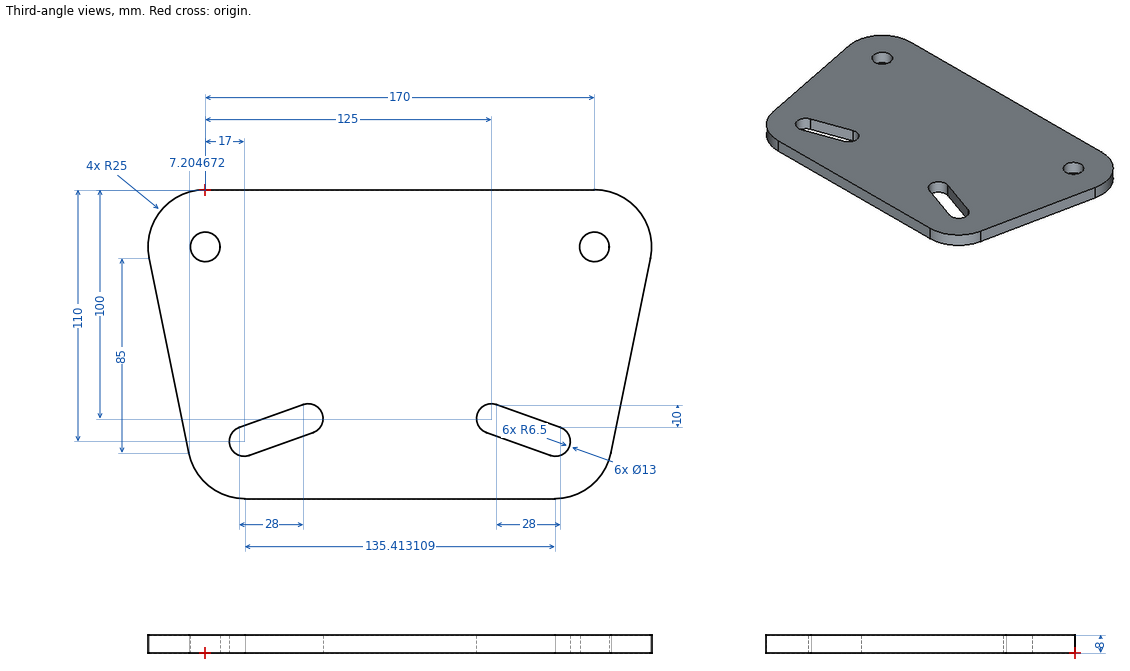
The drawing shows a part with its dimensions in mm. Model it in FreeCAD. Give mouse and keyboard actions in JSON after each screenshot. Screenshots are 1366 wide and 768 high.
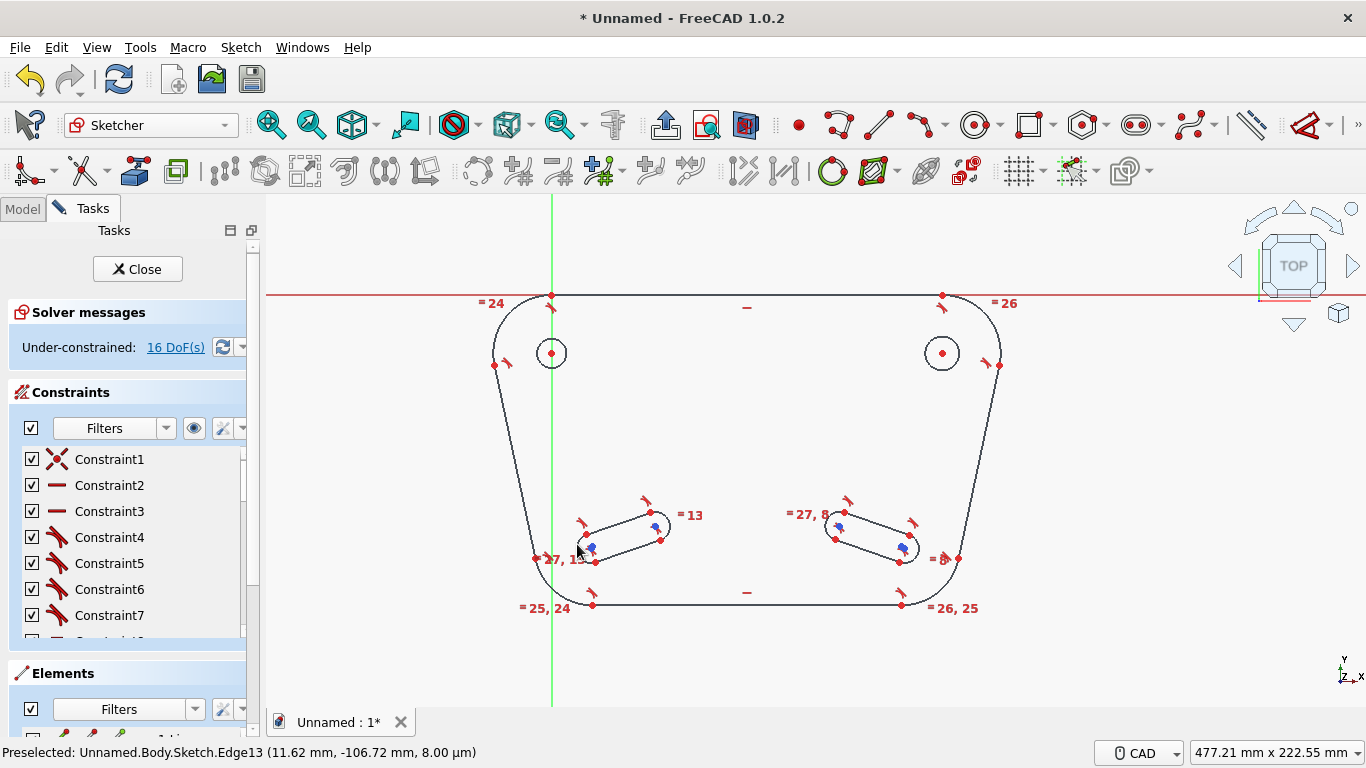
{"action": "left_click", "coordinate": [954, 341]}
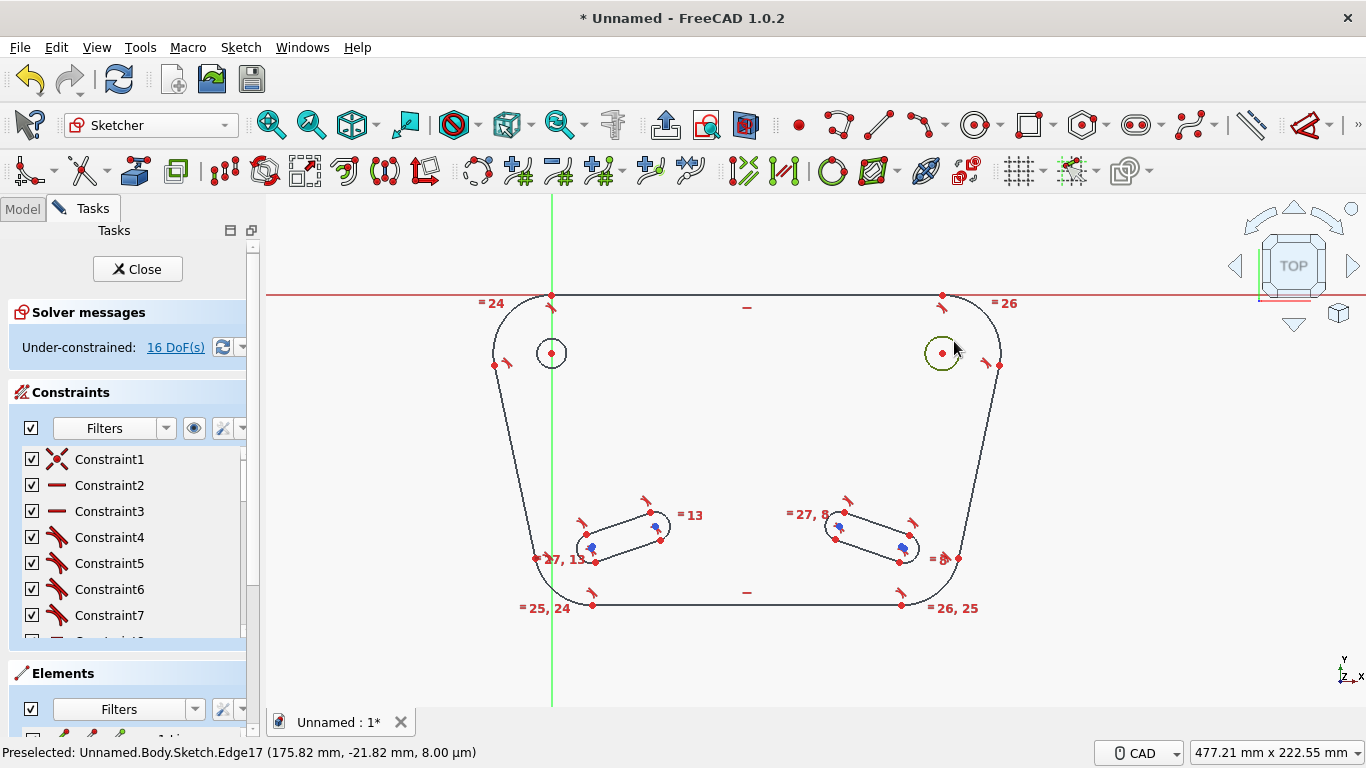
{"action": "scroll", "coordinate": [562, 343], "scroll_direction": "up", "scroll_amount": 2}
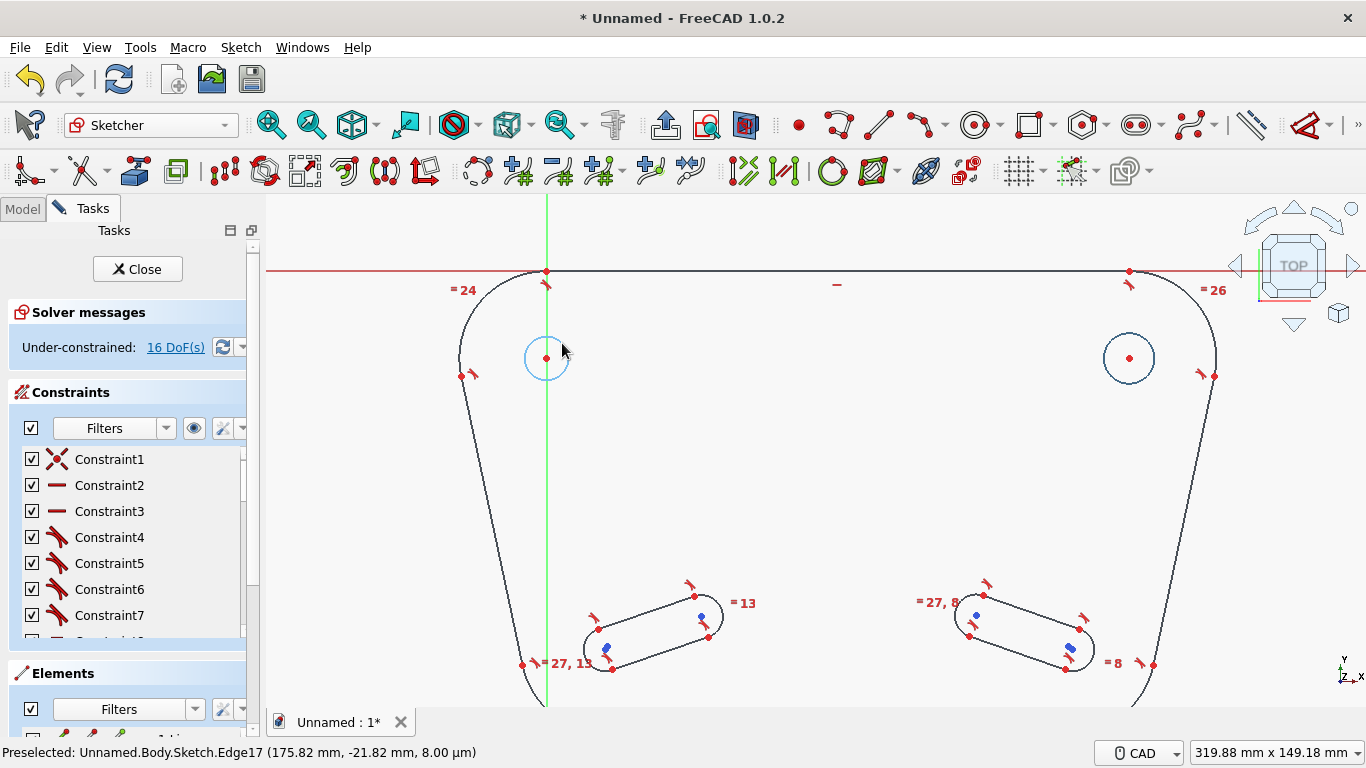
{"action": "left_click", "coordinate": [562, 343]}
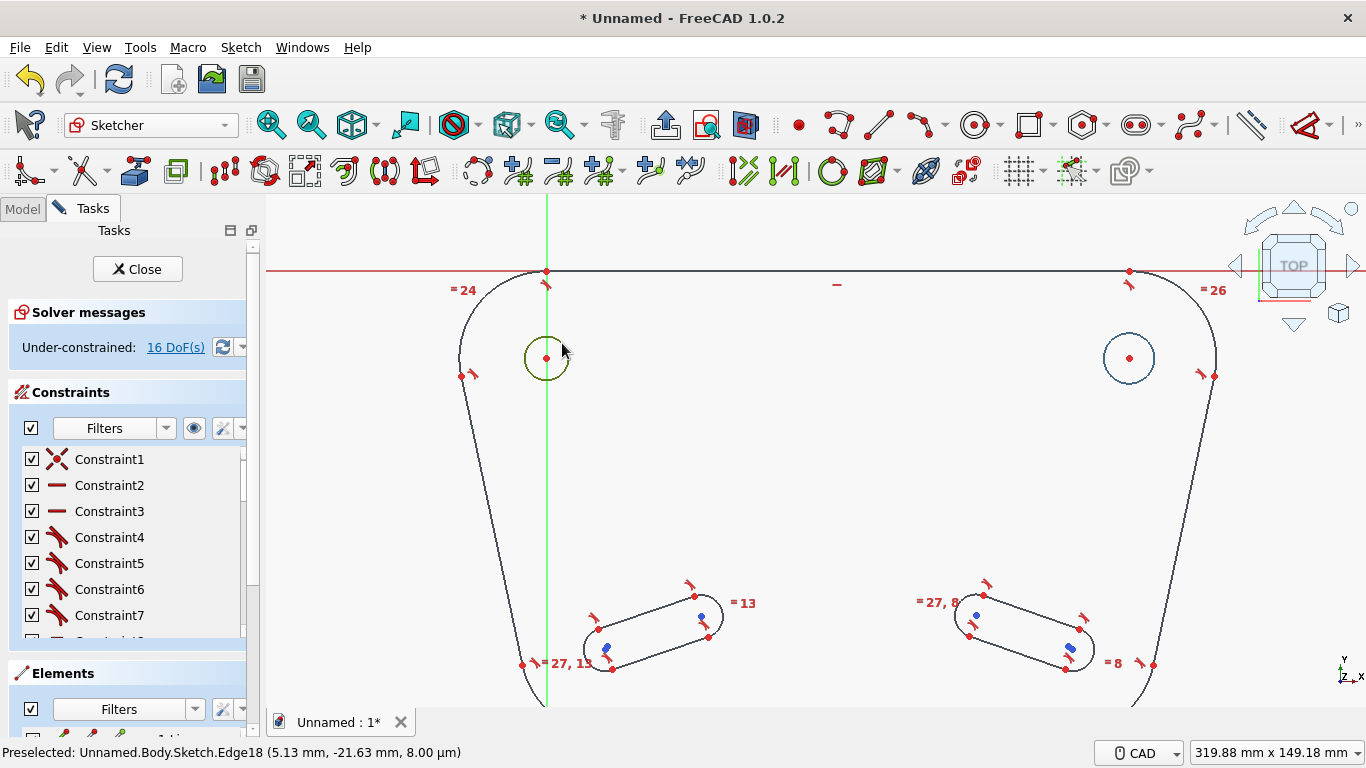
{"action": "key", "text": "e"}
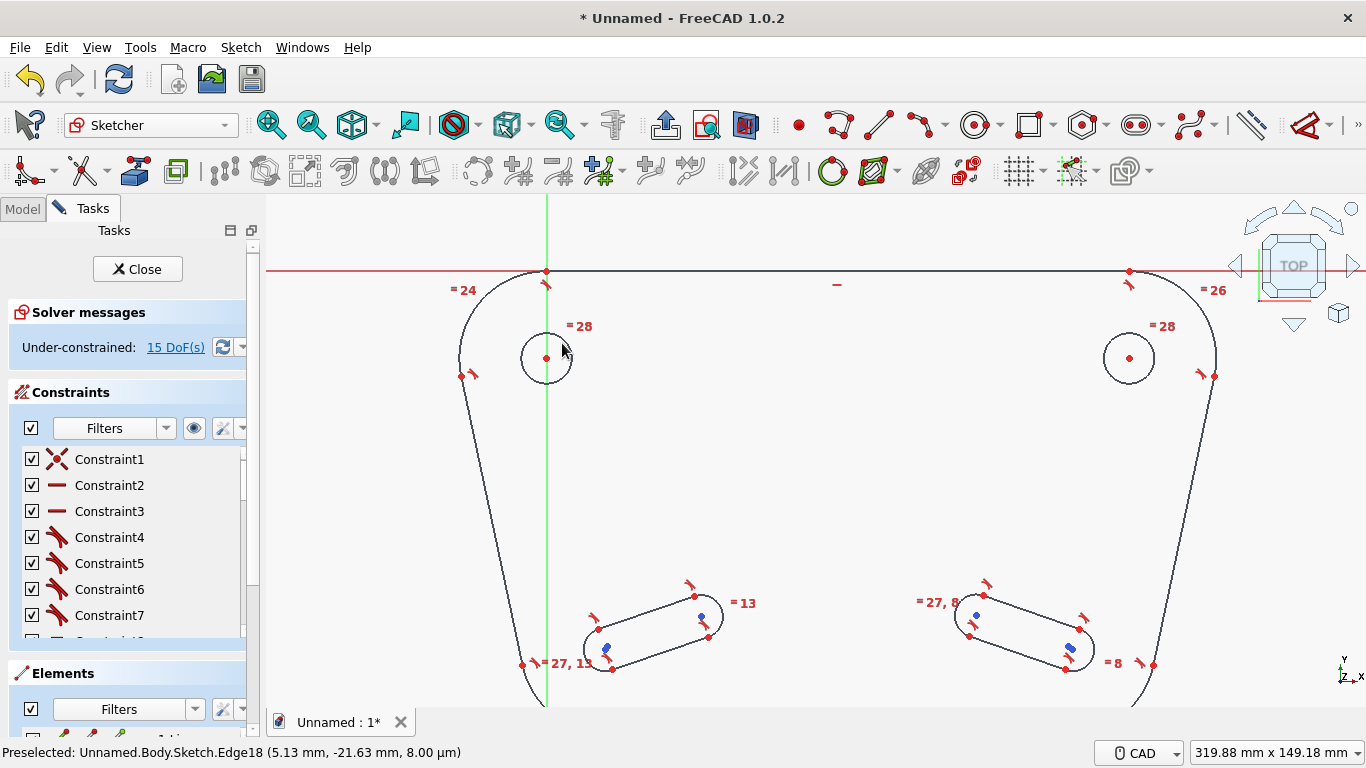
{"action": "left_click", "coordinate": [1306, 126]}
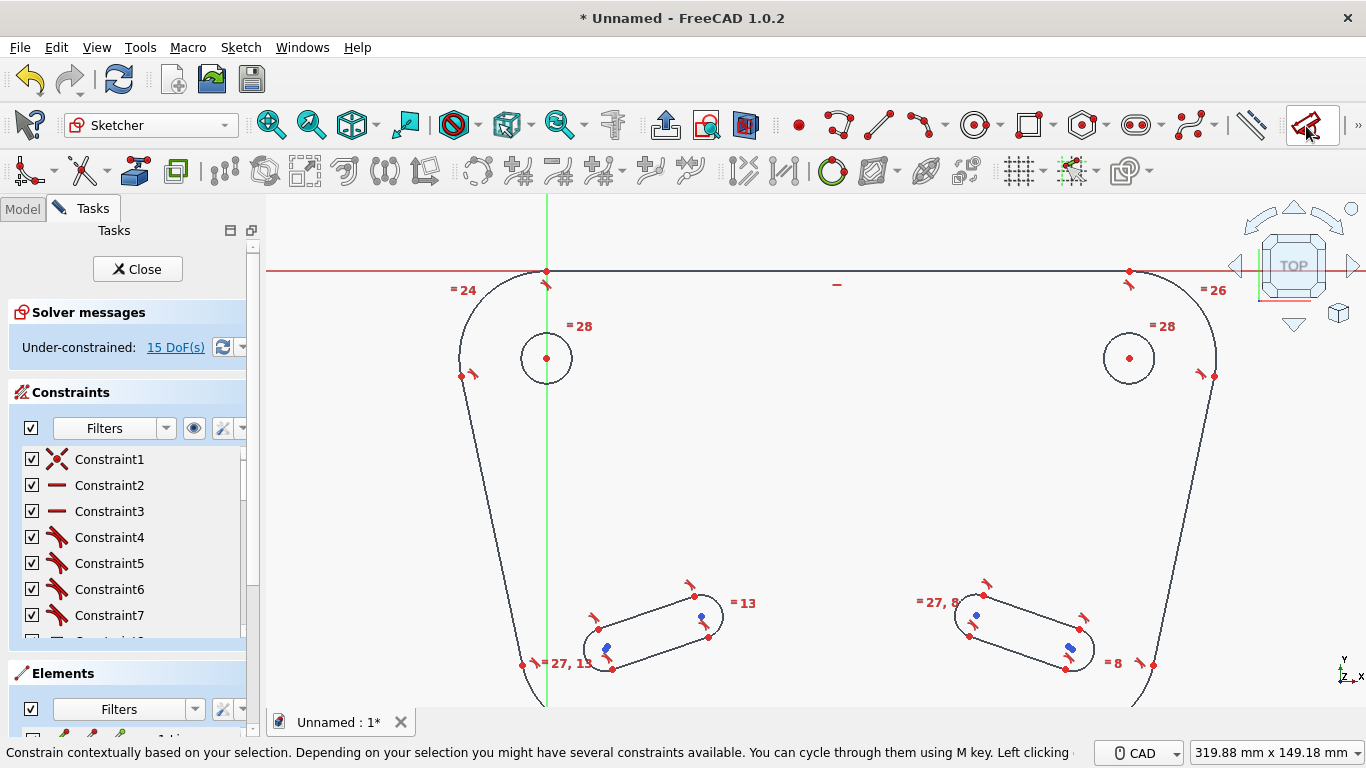
{"action": "left_click", "coordinate": [502, 283]}
{"action": "left_click", "coordinate": [486, 255]}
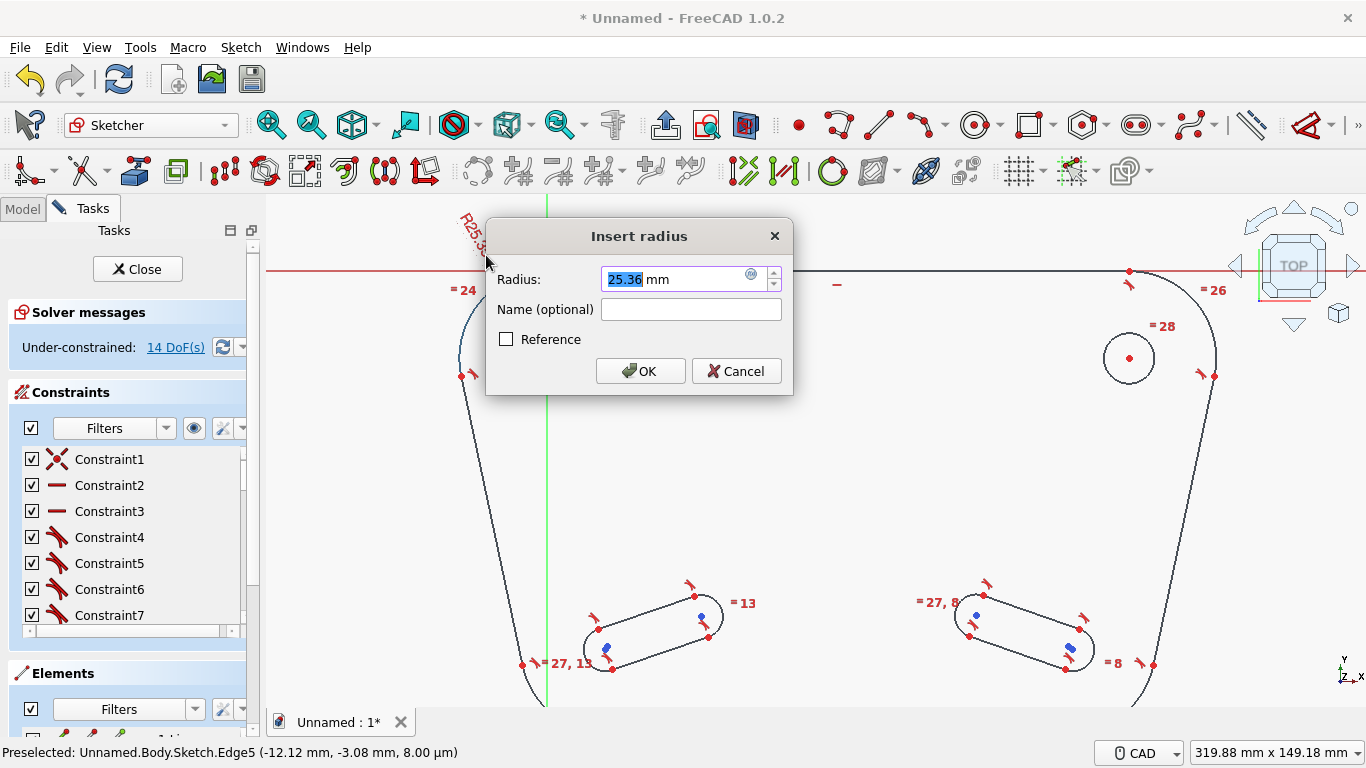
{"action": "type", "text": "25"}
{"action": "key", "text": "Return"}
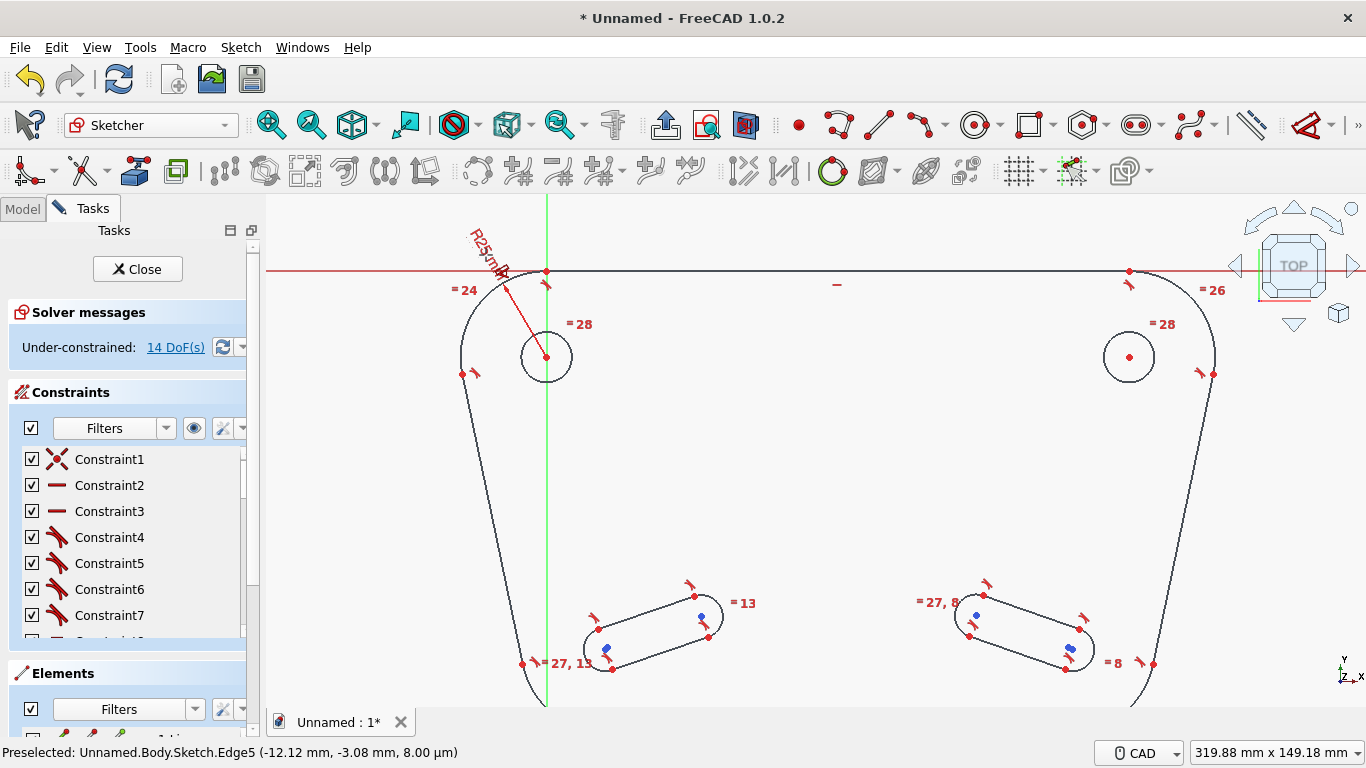
{"action": "scroll", "coordinate": [964, 598], "scroll_direction": "up", "scroll_amount": 3}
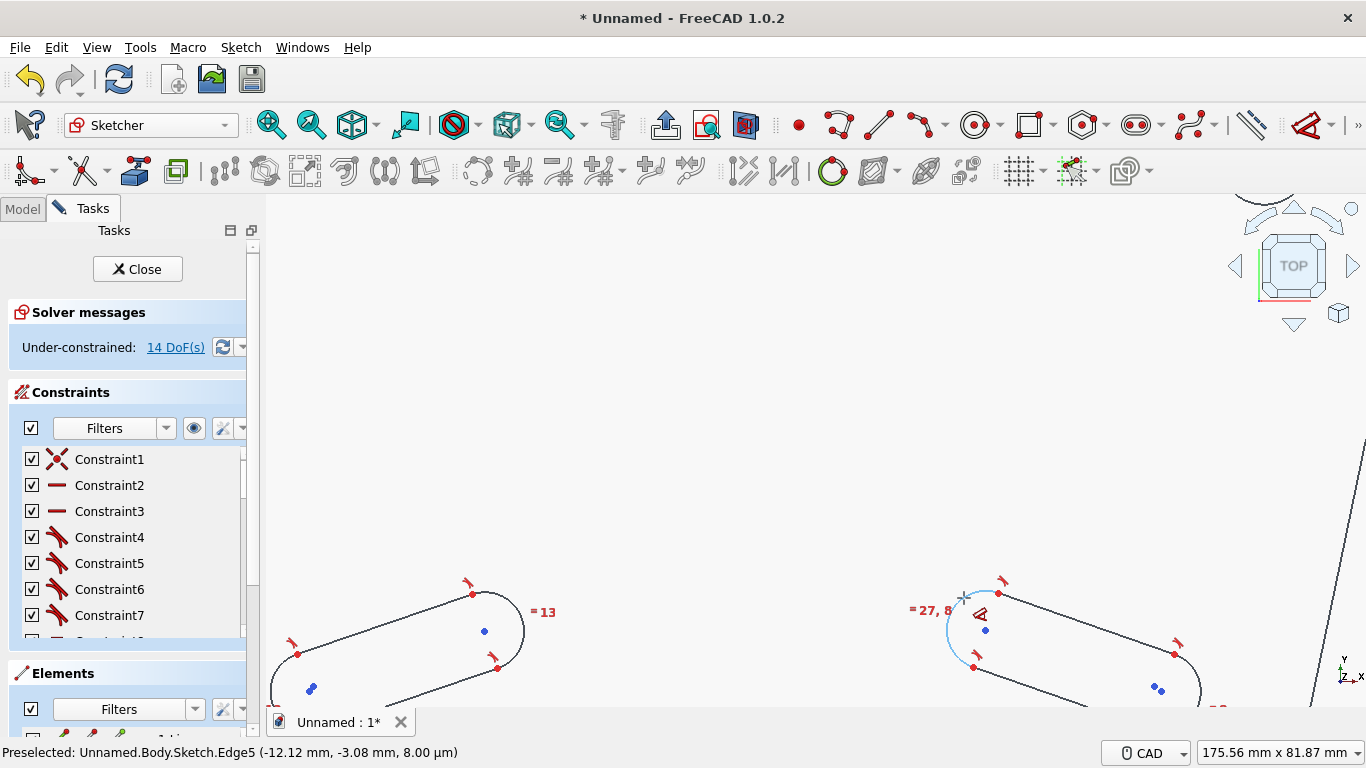
{"action": "left_click", "coordinate": [964, 598]}
{"action": "left_click", "coordinate": [946, 572]}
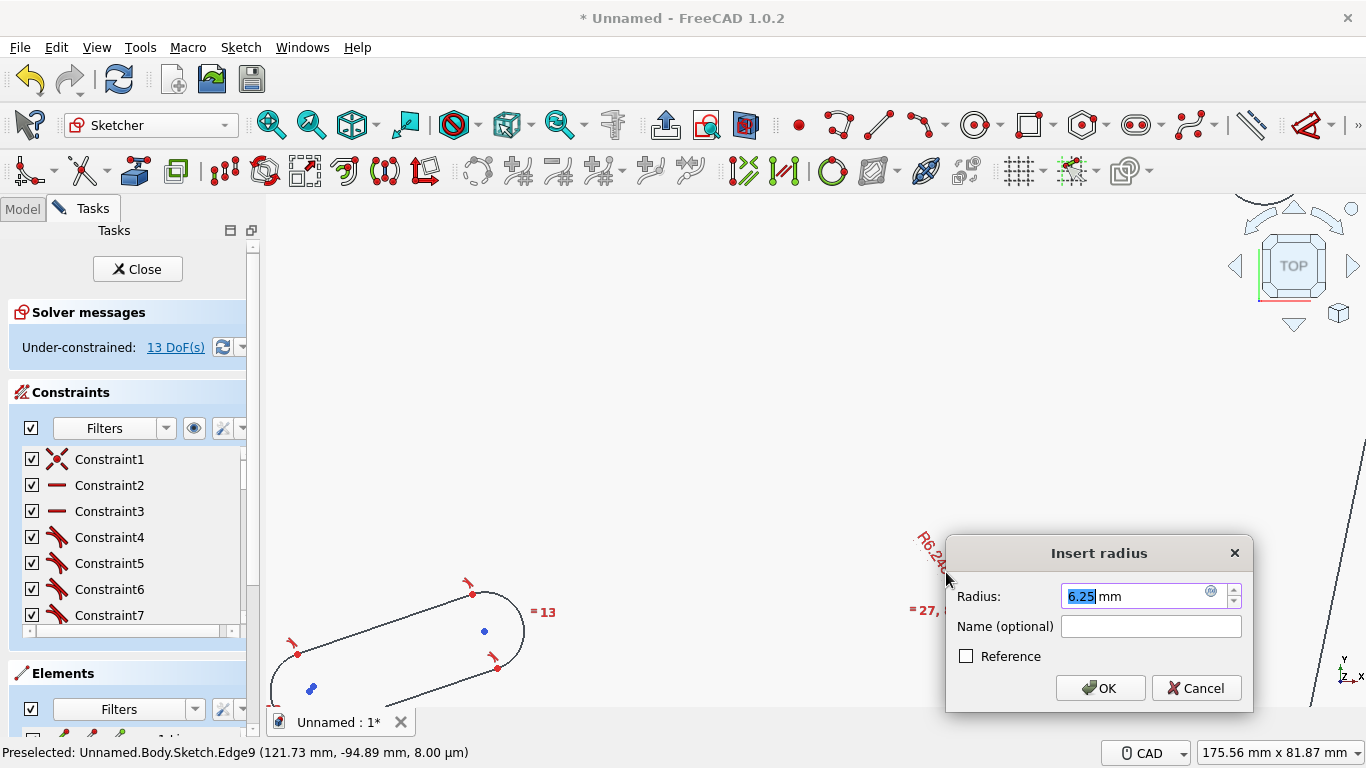
{"action": "type", "text": "6.5"}
{"action": "key", "text": "Return"}